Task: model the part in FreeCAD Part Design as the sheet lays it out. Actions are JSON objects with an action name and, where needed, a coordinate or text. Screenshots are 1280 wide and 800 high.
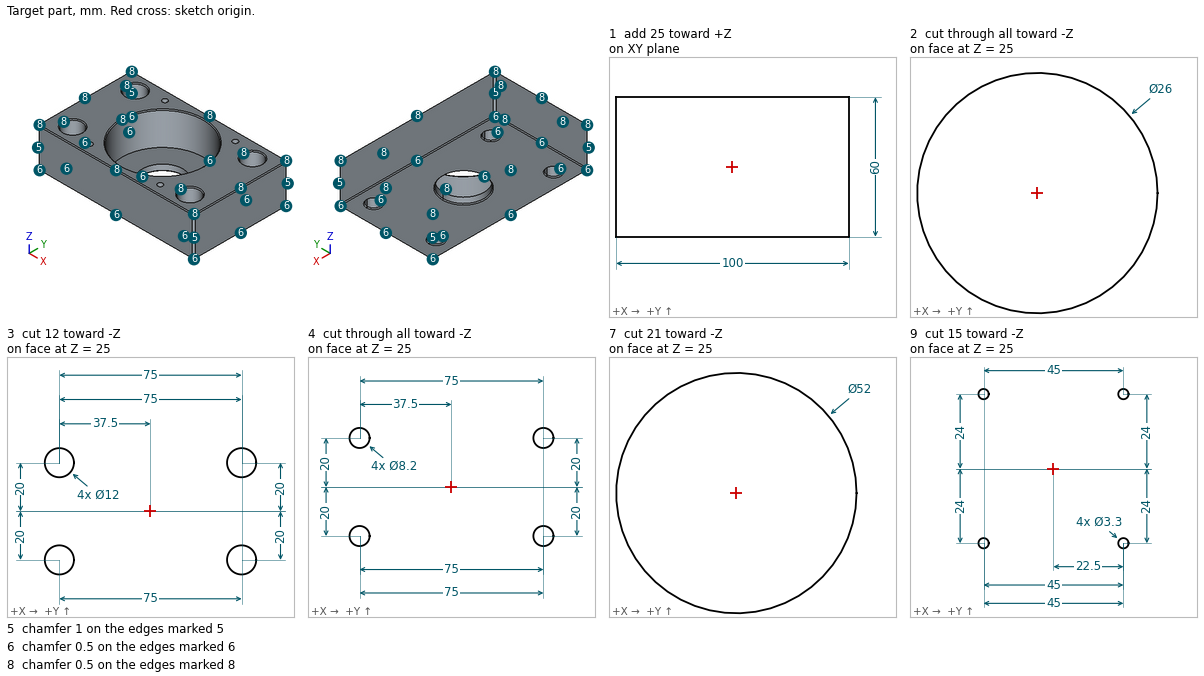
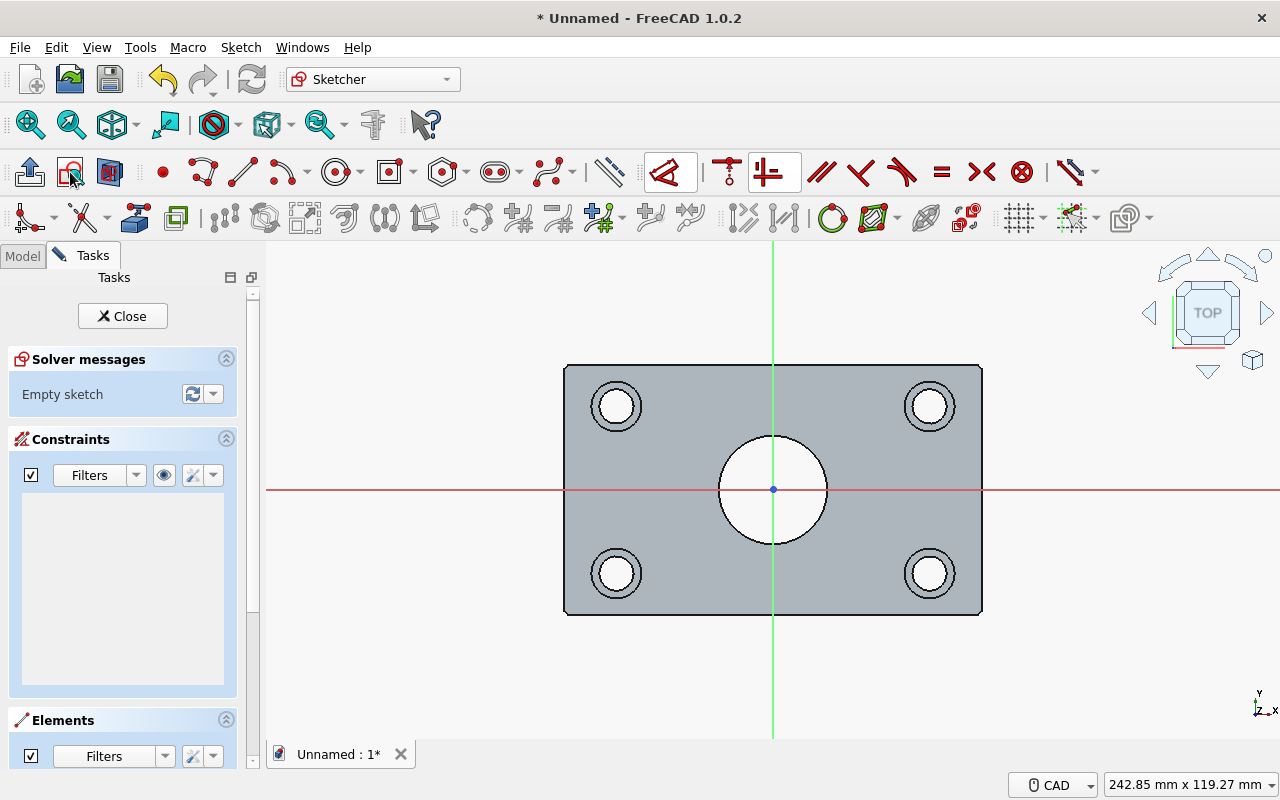
{"action": "scroll", "coordinate": [912, 490], "scroll_direction": "up", "scroll_amount": 2}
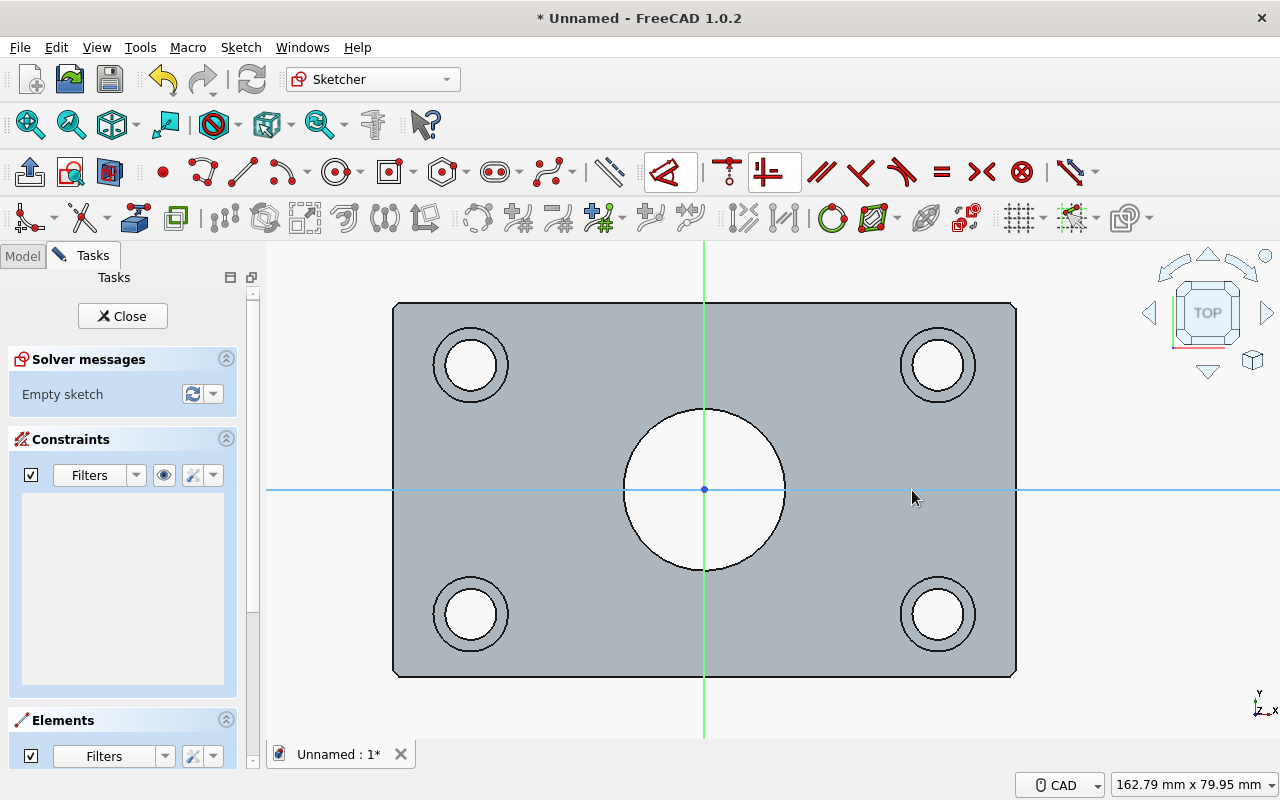
{"action": "left_click", "coordinate": [336, 172]}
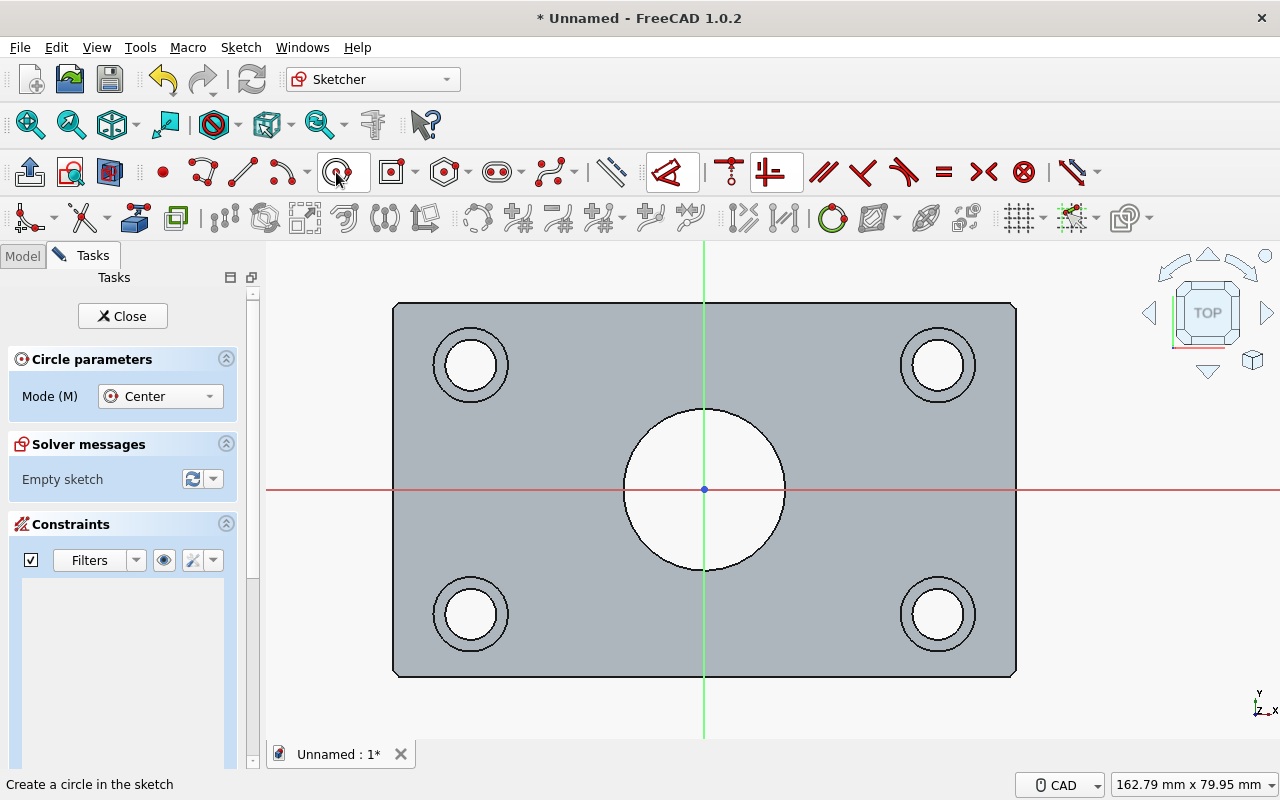
{"action": "left_click", "coordinate": [704, 490]}
{"action": "mouse_move", "coordinate": [819, 375]}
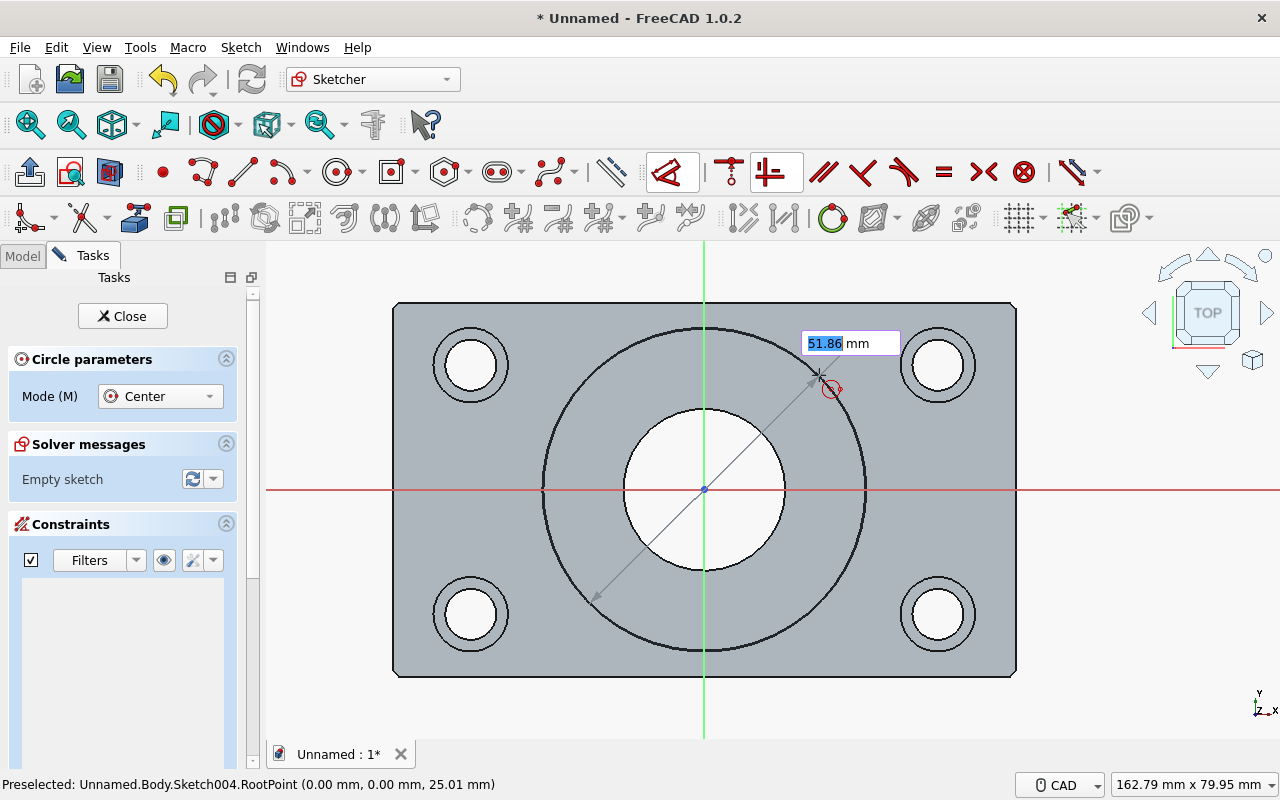
{"action": "type", "text": "52"}
{"action": "key", "text": "Return"}
{"action": "key", "text": "Escape"}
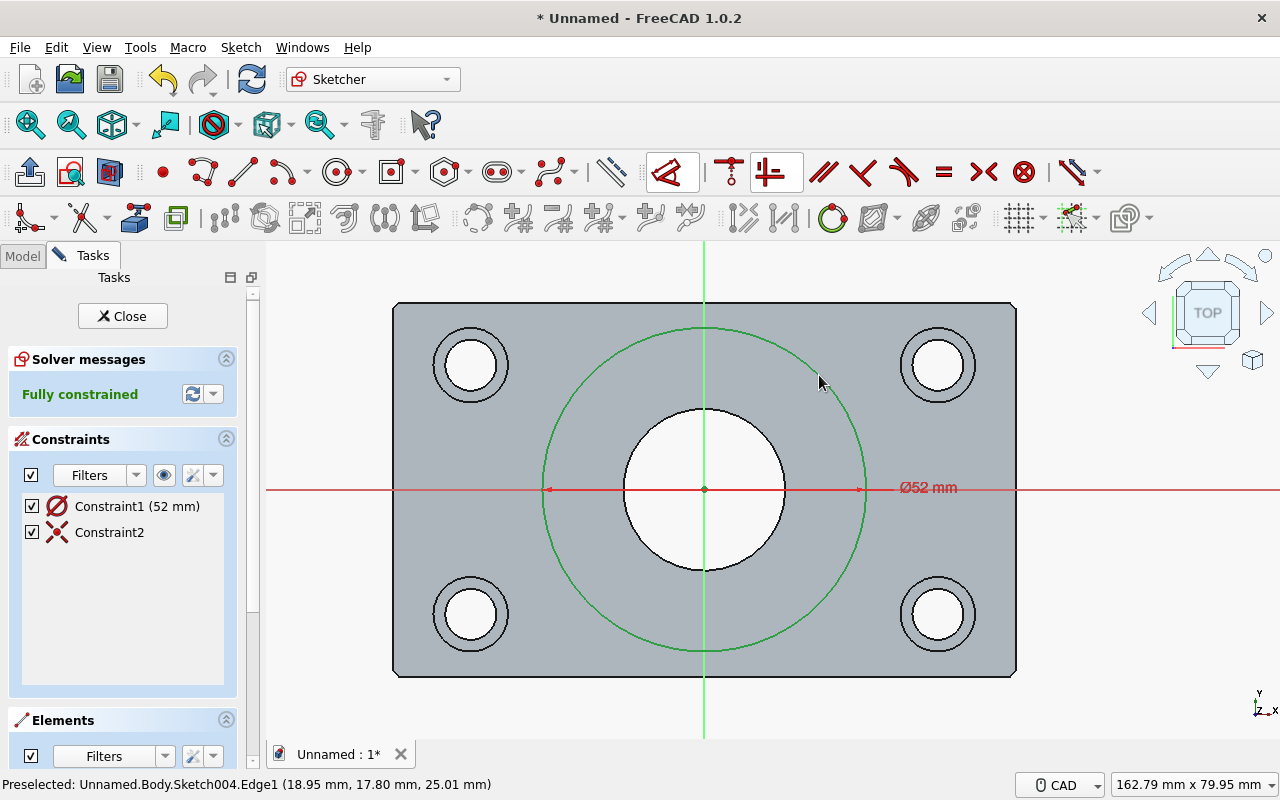
{"action": "left_click", "coordinate": [123, 316]}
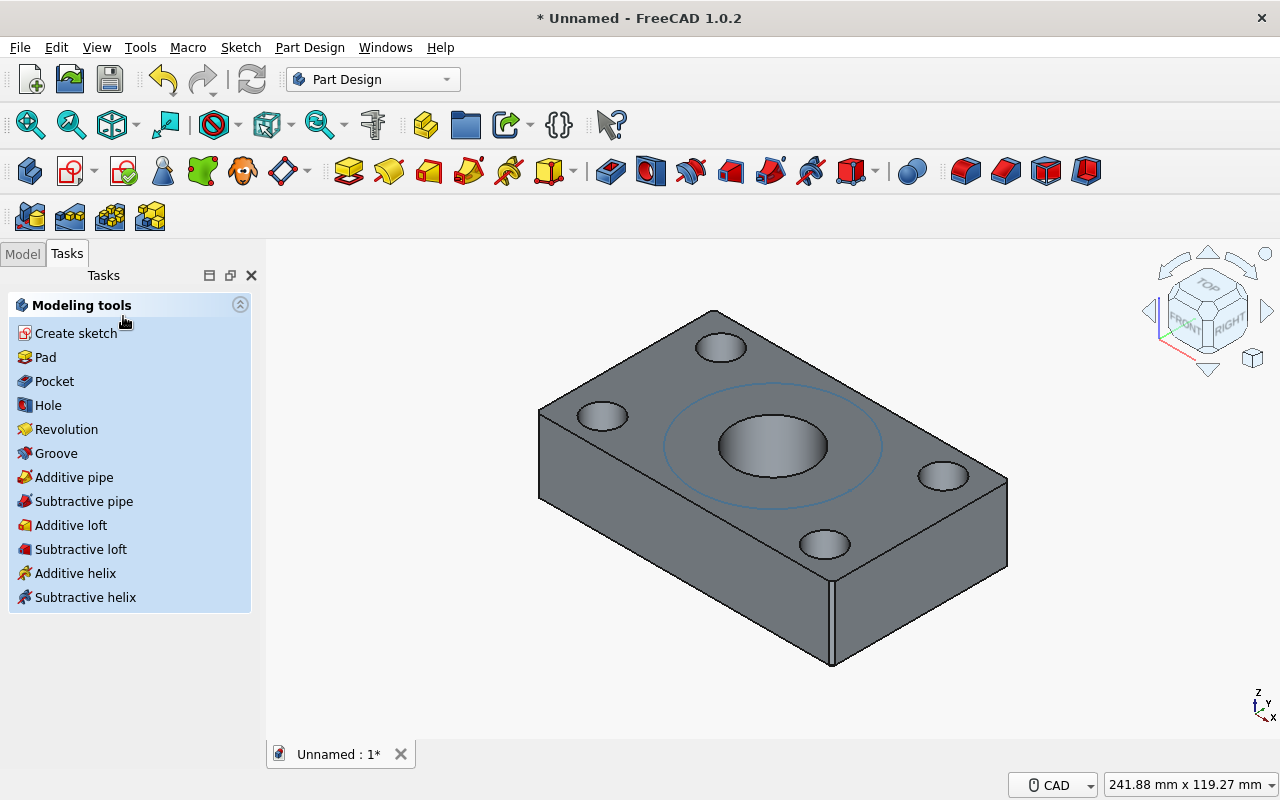
{"action": "left_click", "coordinate": [612, 172]}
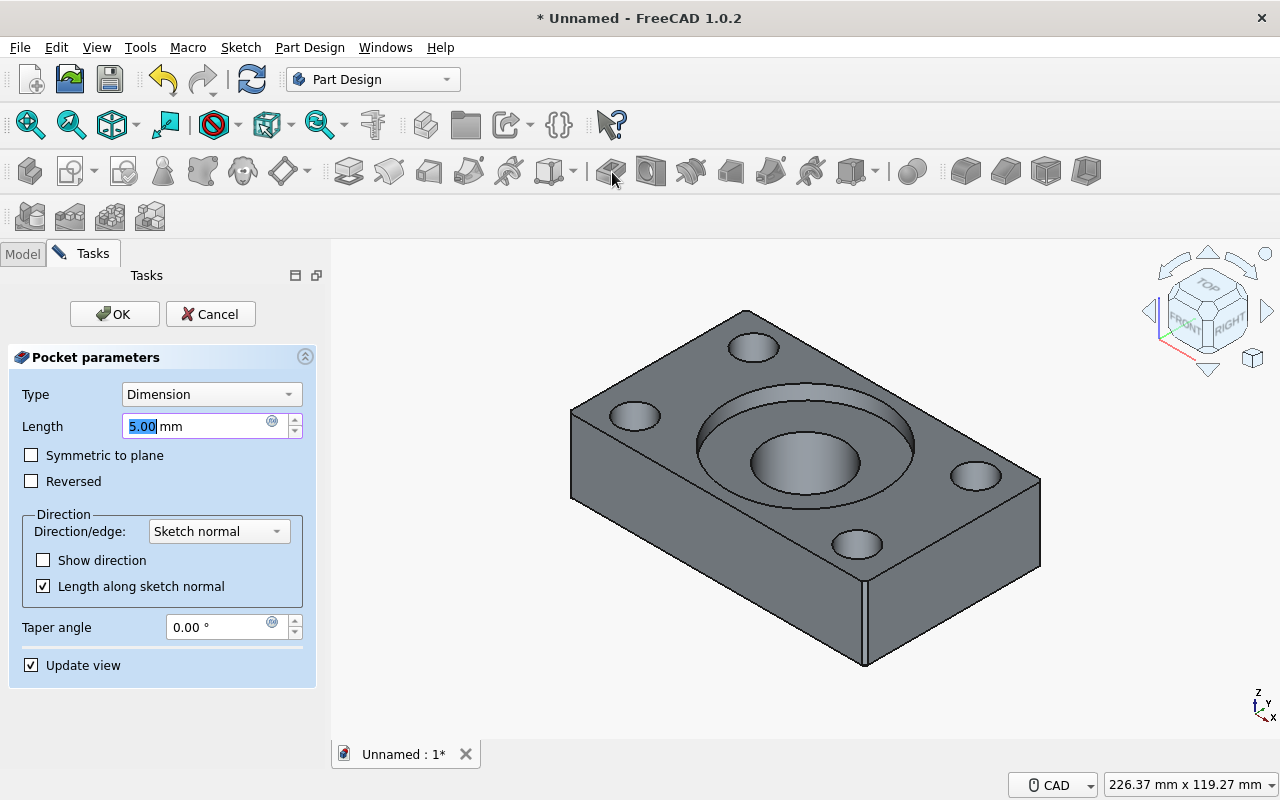
{"action": "type", "text": "21"}
{"action": "key", "text": "Tab"}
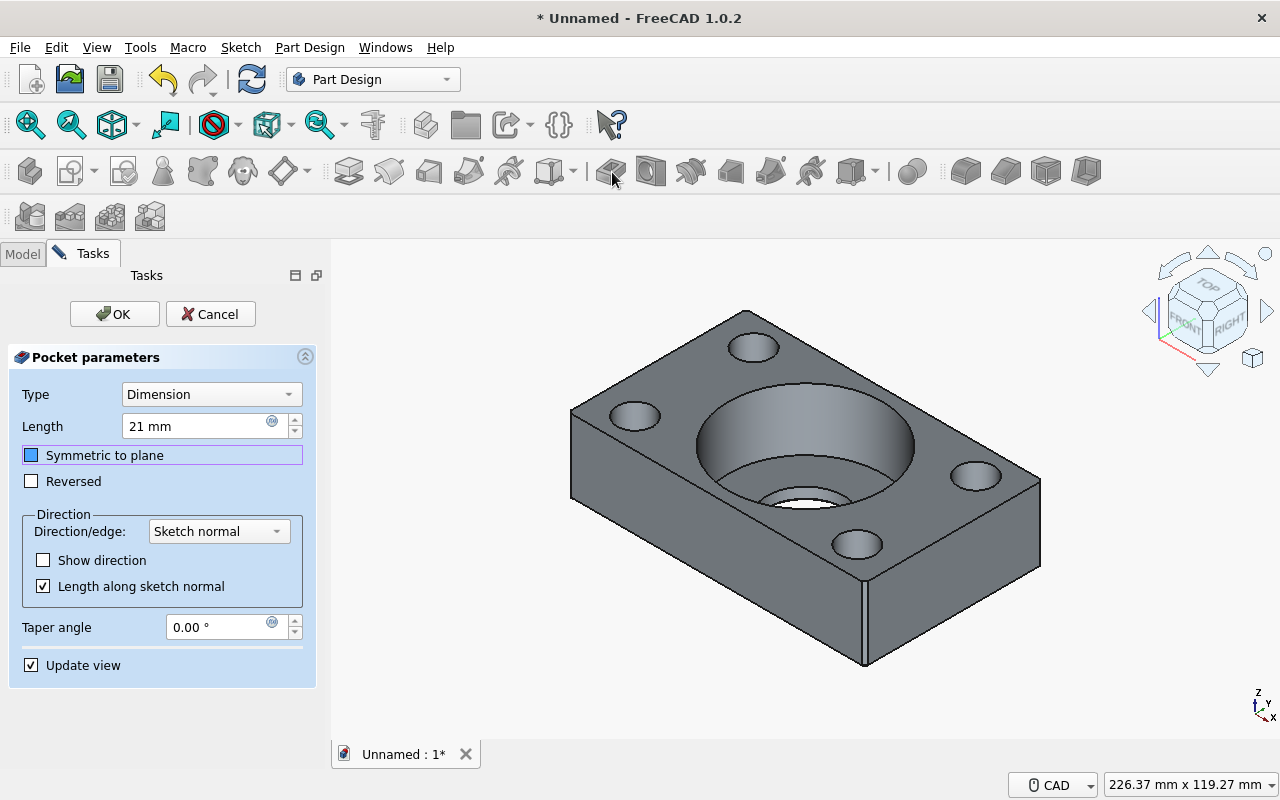
{"action": "left_click", "coordinate": [115, 314]}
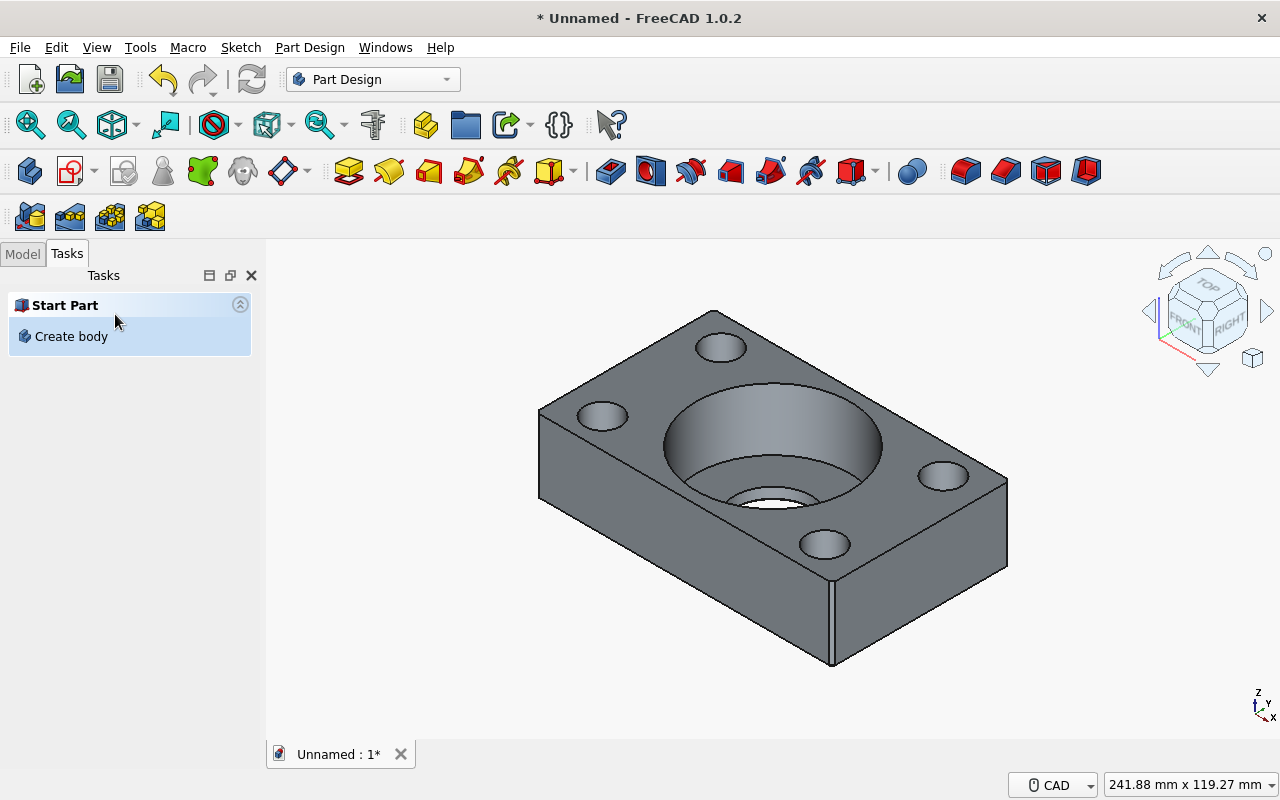
{"action": "left_click", "coordinate": [646, 372]}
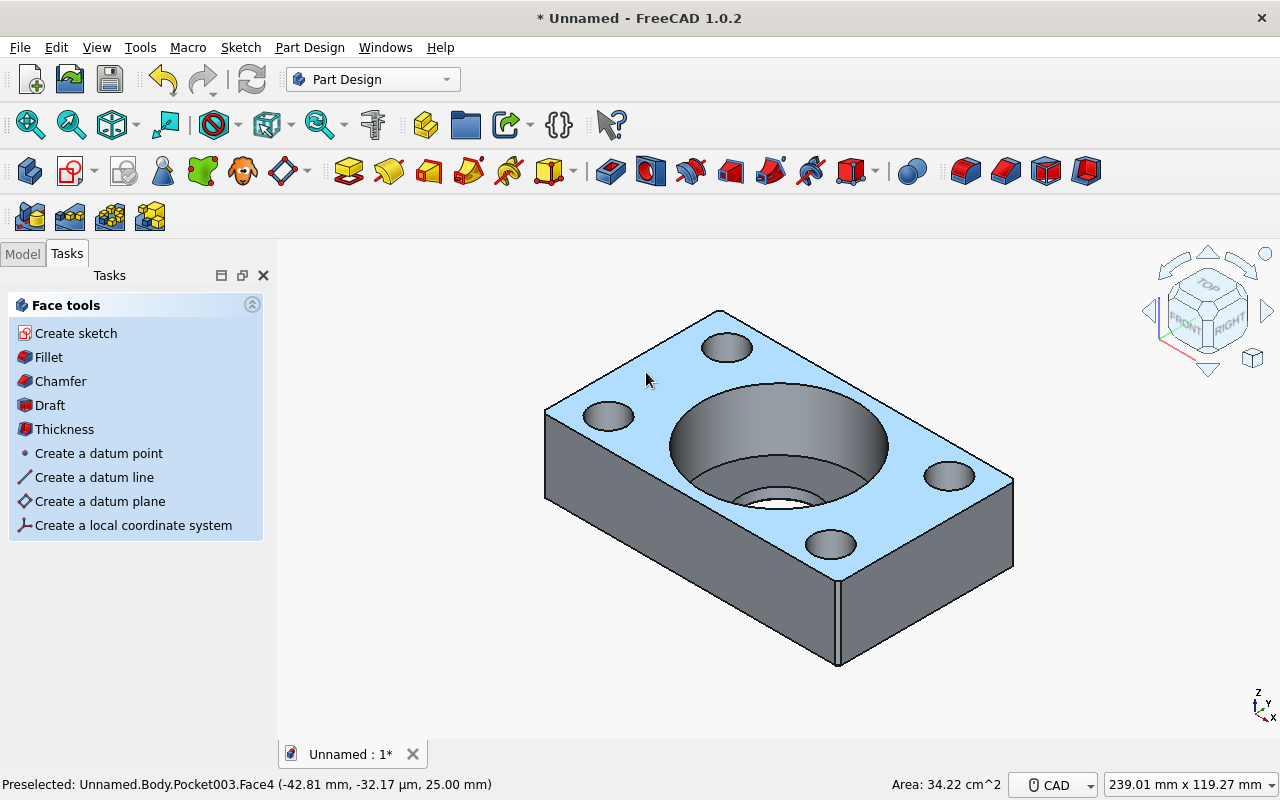
{"action": "left_click", "coordinate": [1006, 172]}